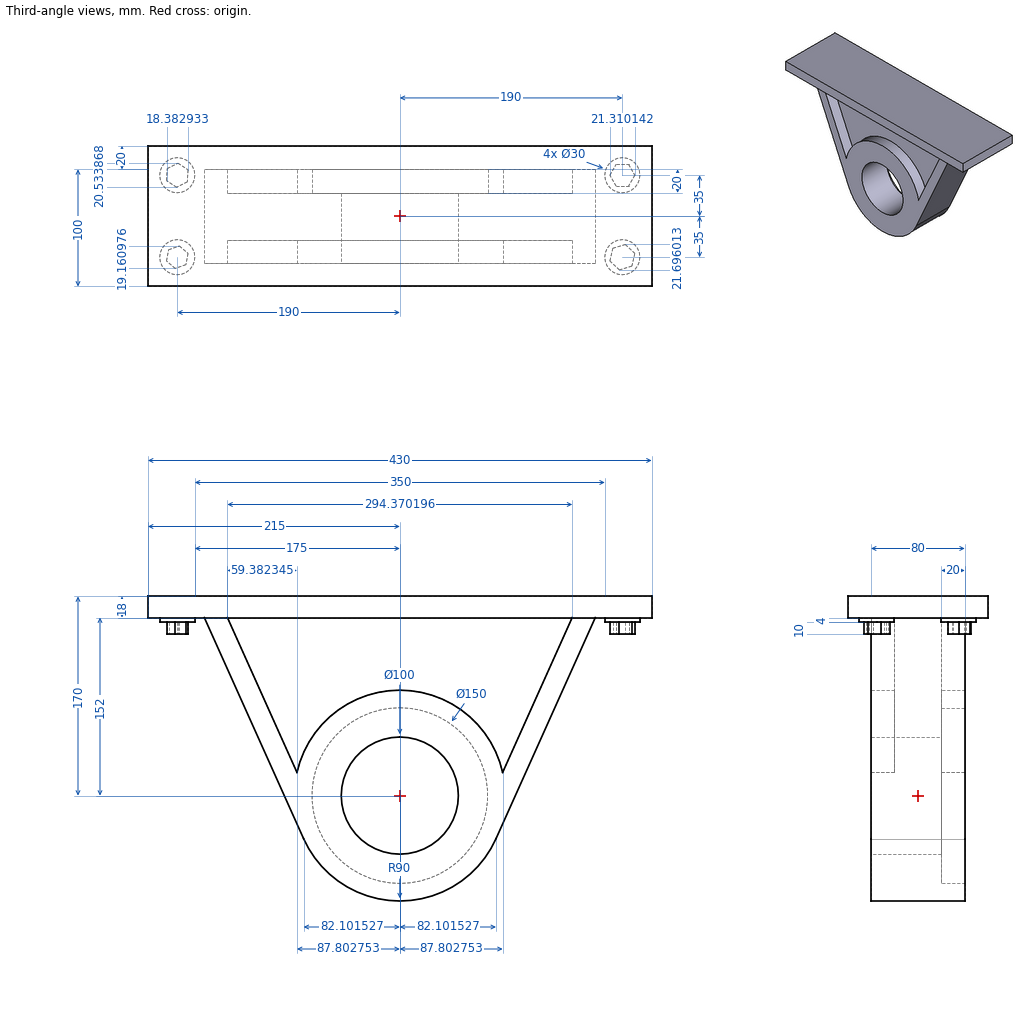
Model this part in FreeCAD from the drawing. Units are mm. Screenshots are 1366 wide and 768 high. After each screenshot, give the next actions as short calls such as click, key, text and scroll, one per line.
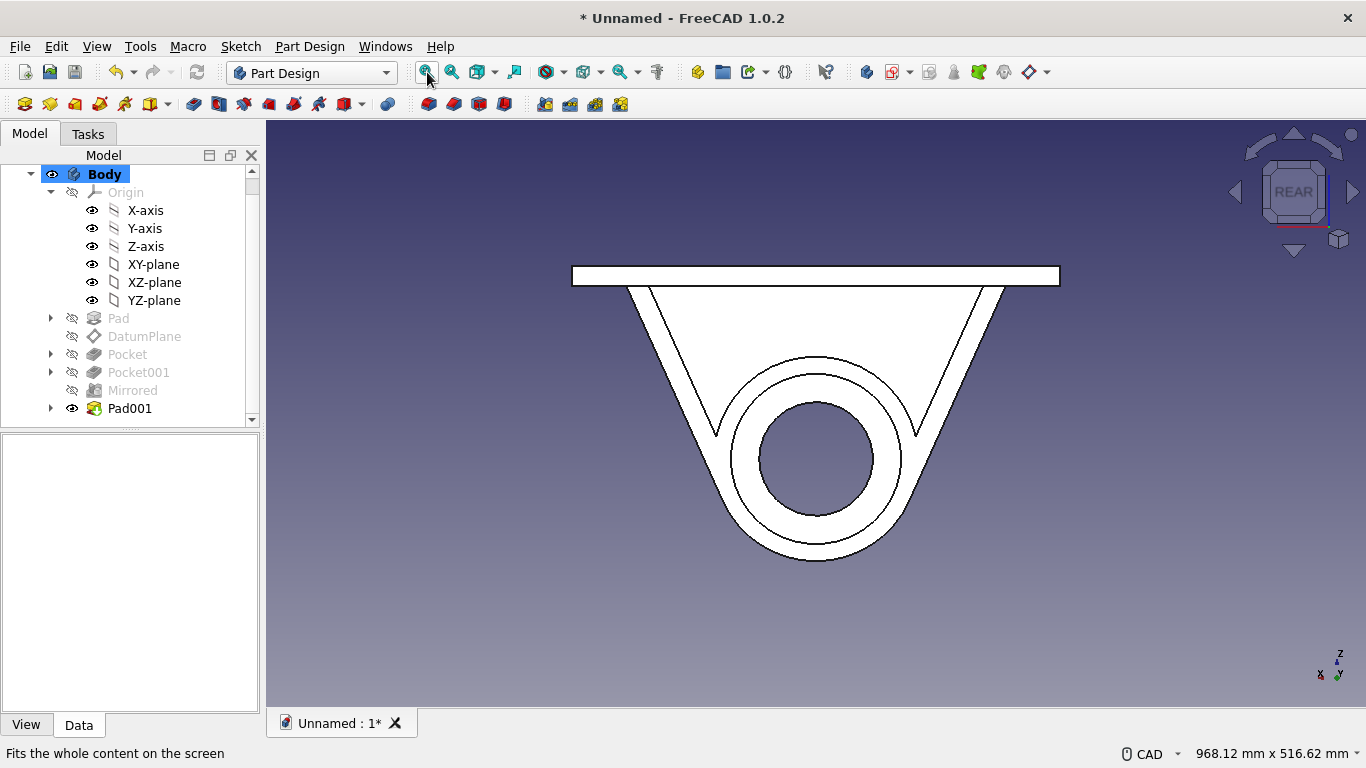
key(5)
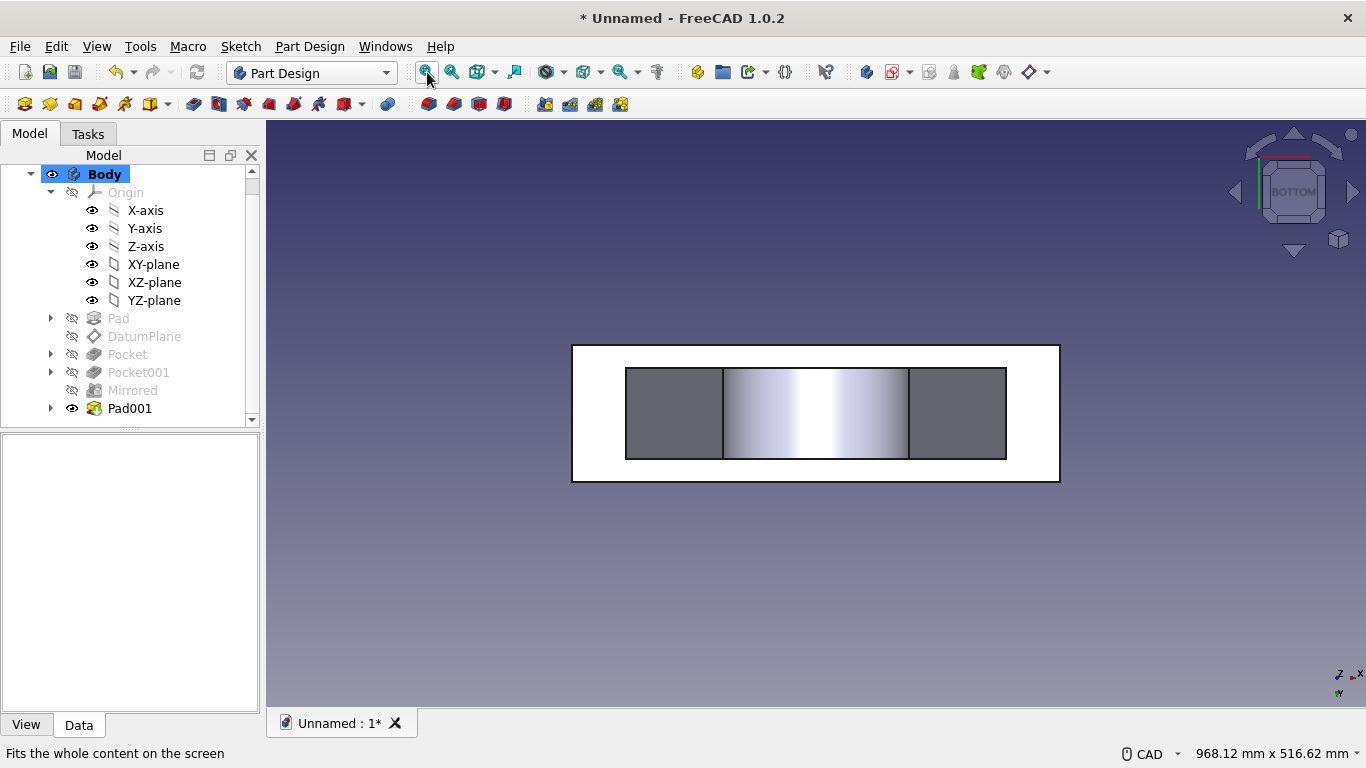
click(427, 72)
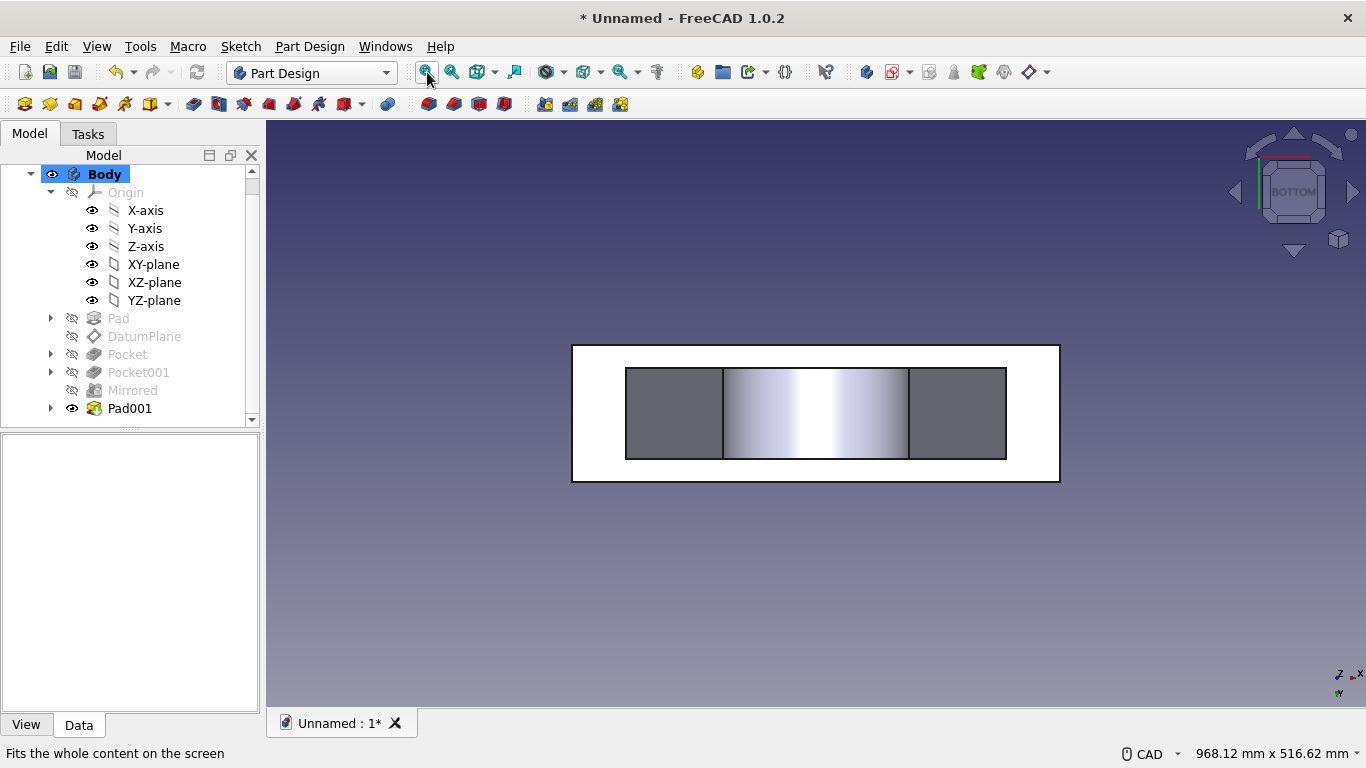
click(1025, 451)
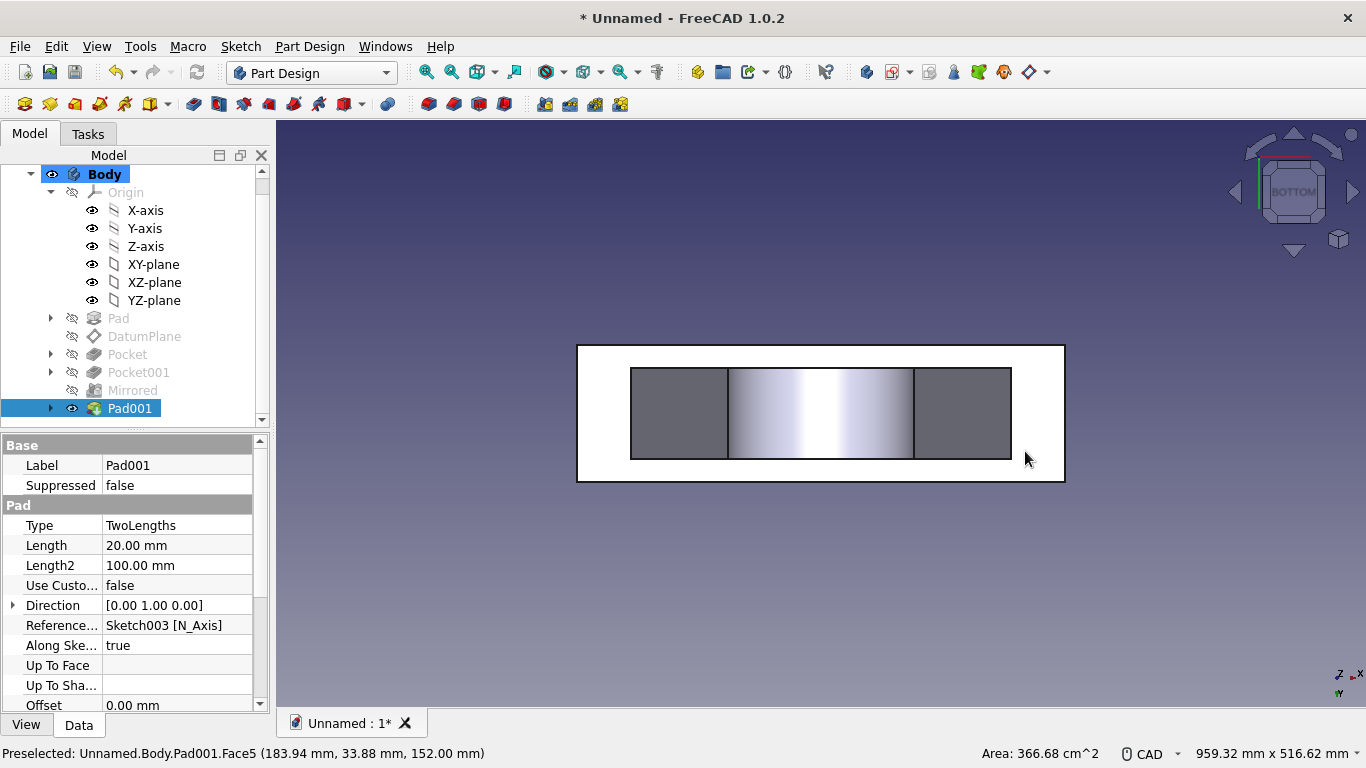
click(892, 72)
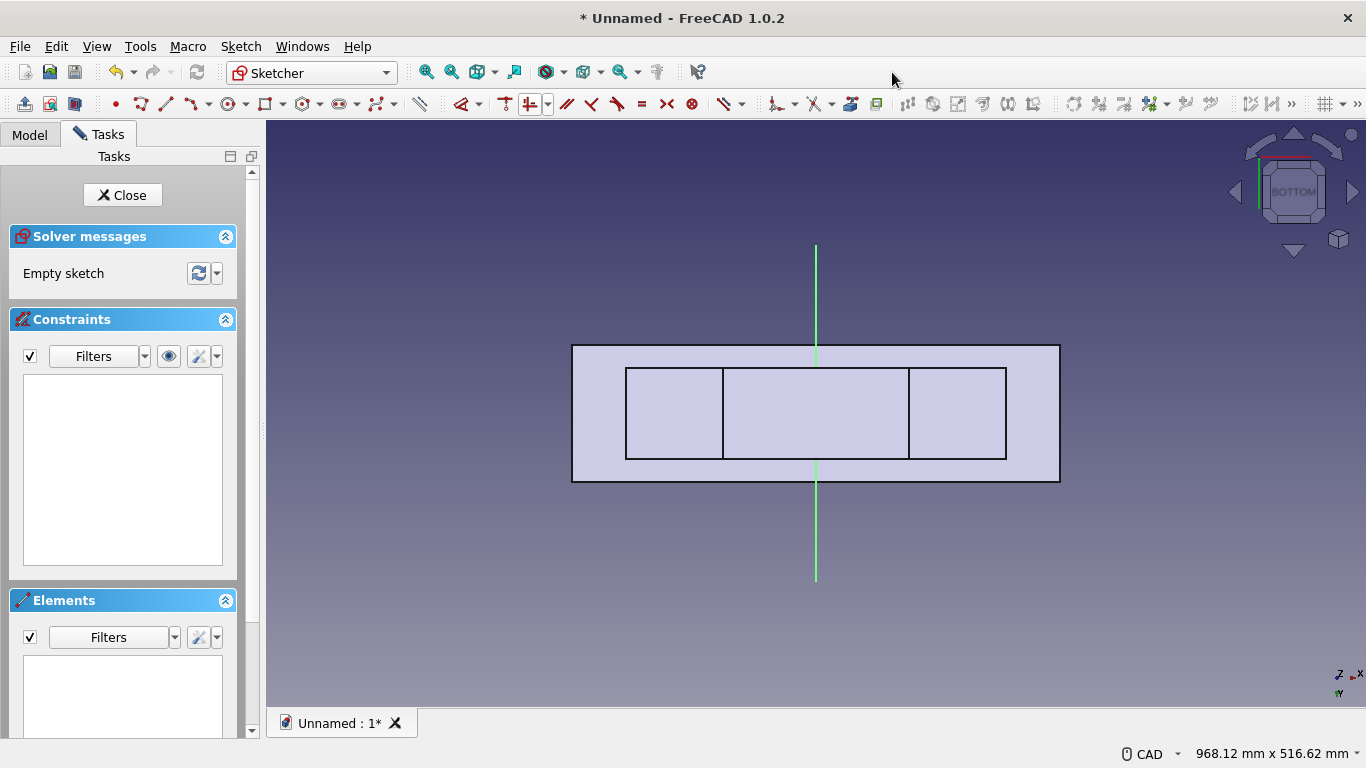
scroll(955, 414, up, 2)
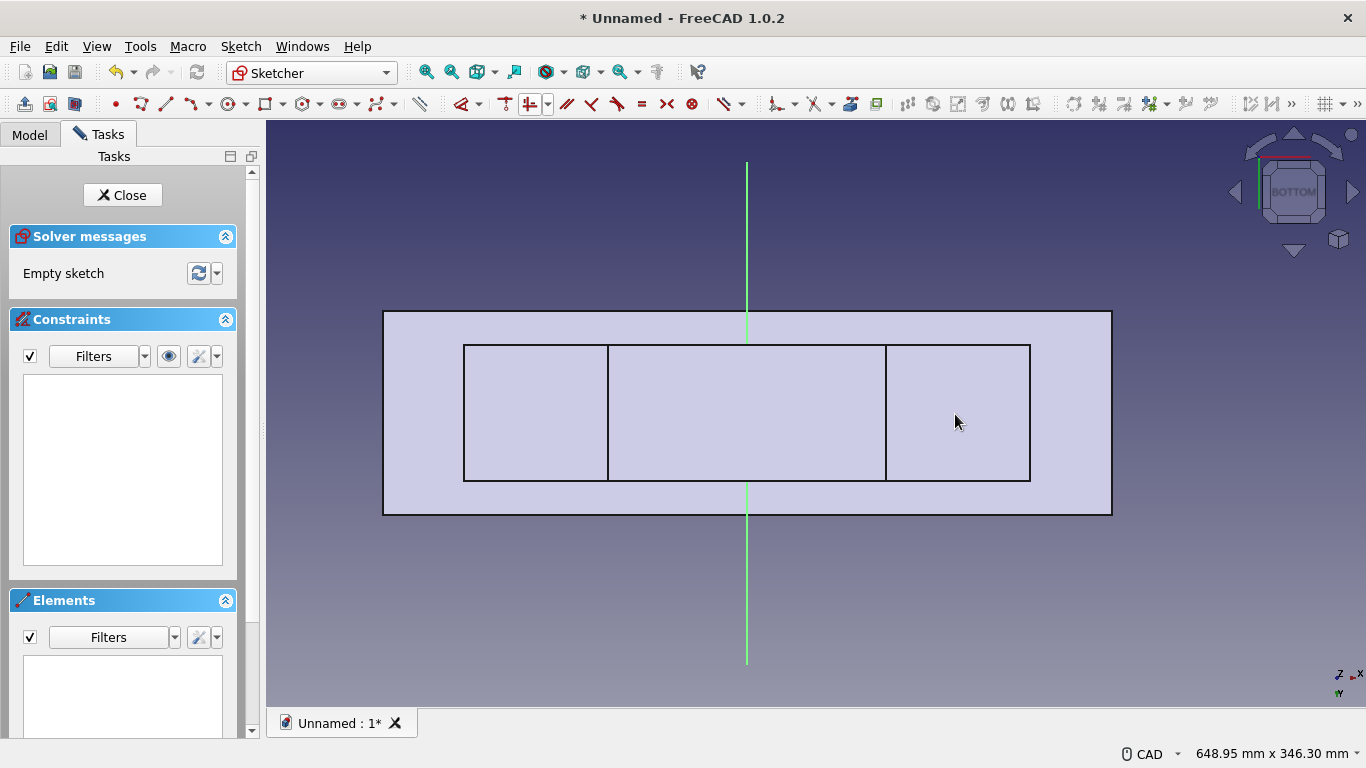
click(228, 104)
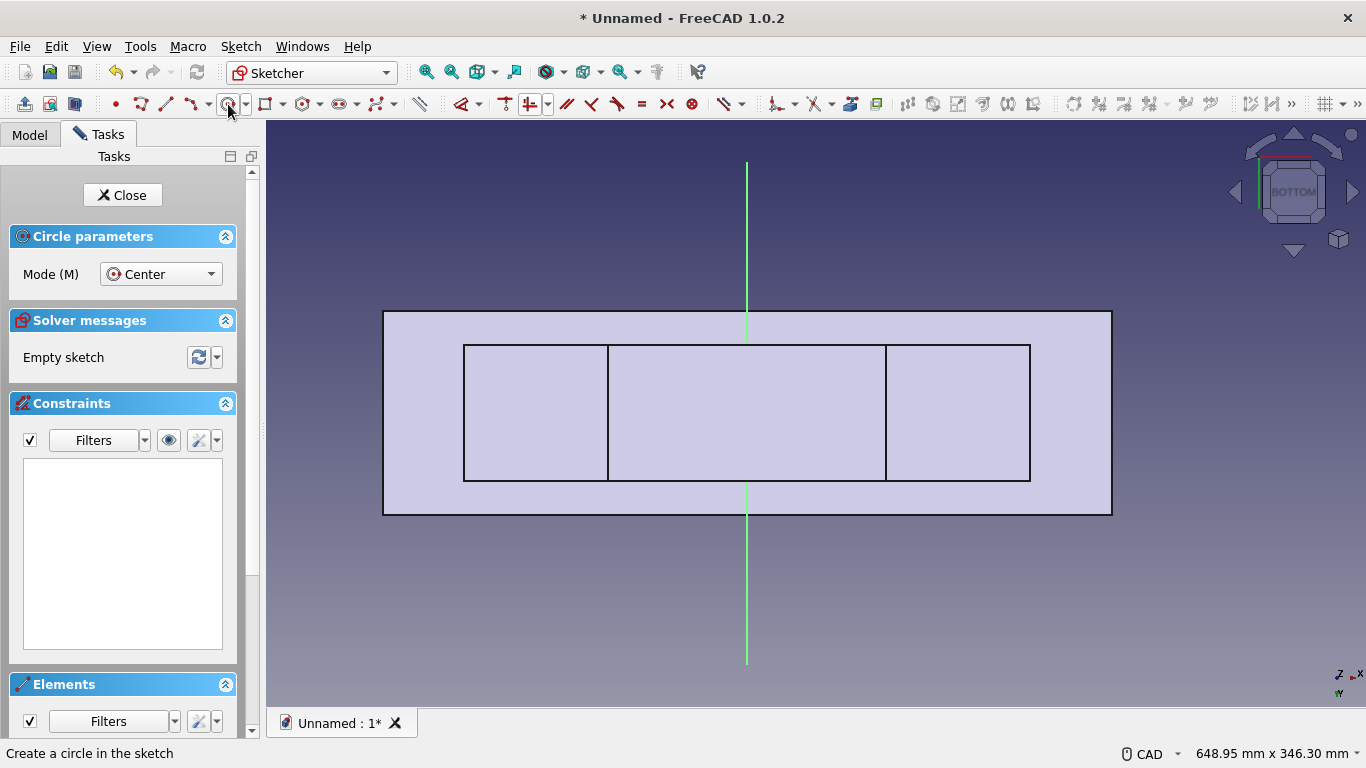
click(1069, 472)
click(1087, 454)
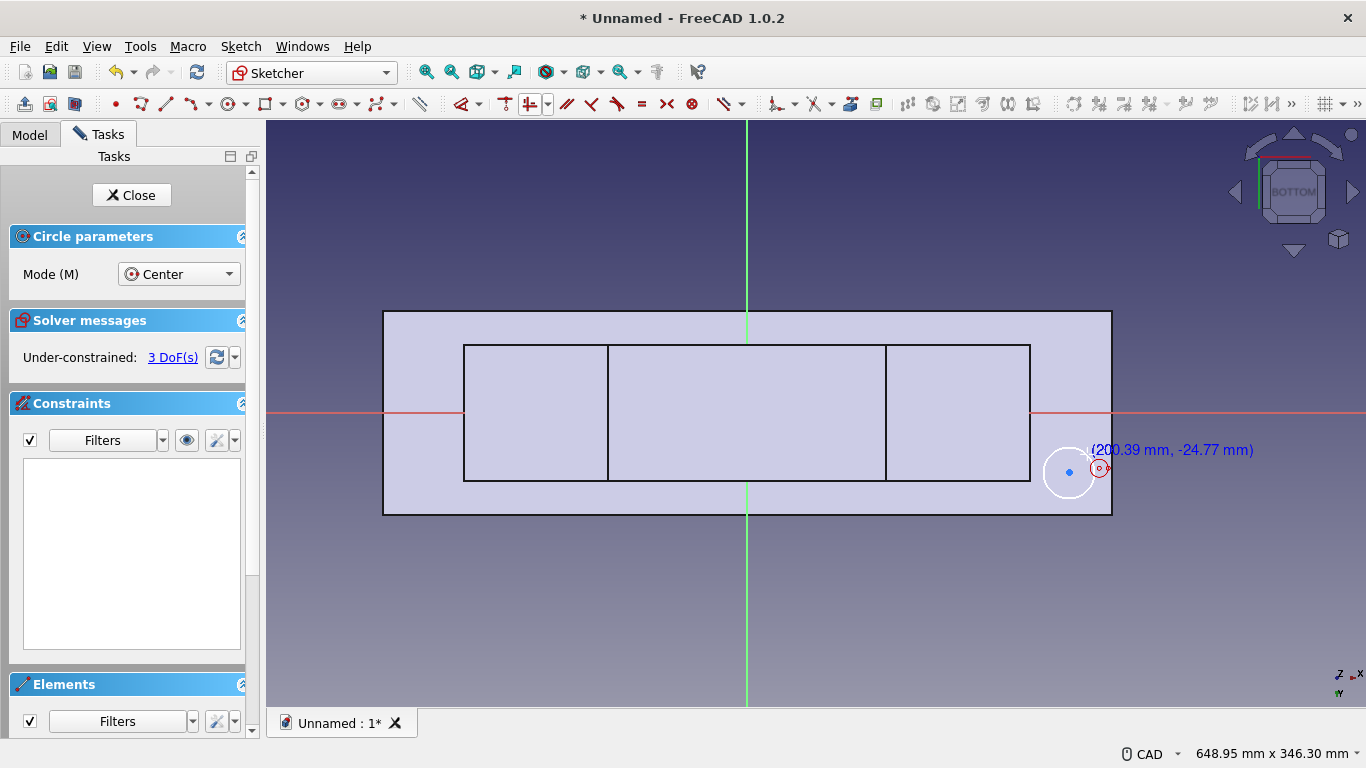
click(1069, 354)
click(1087, 336)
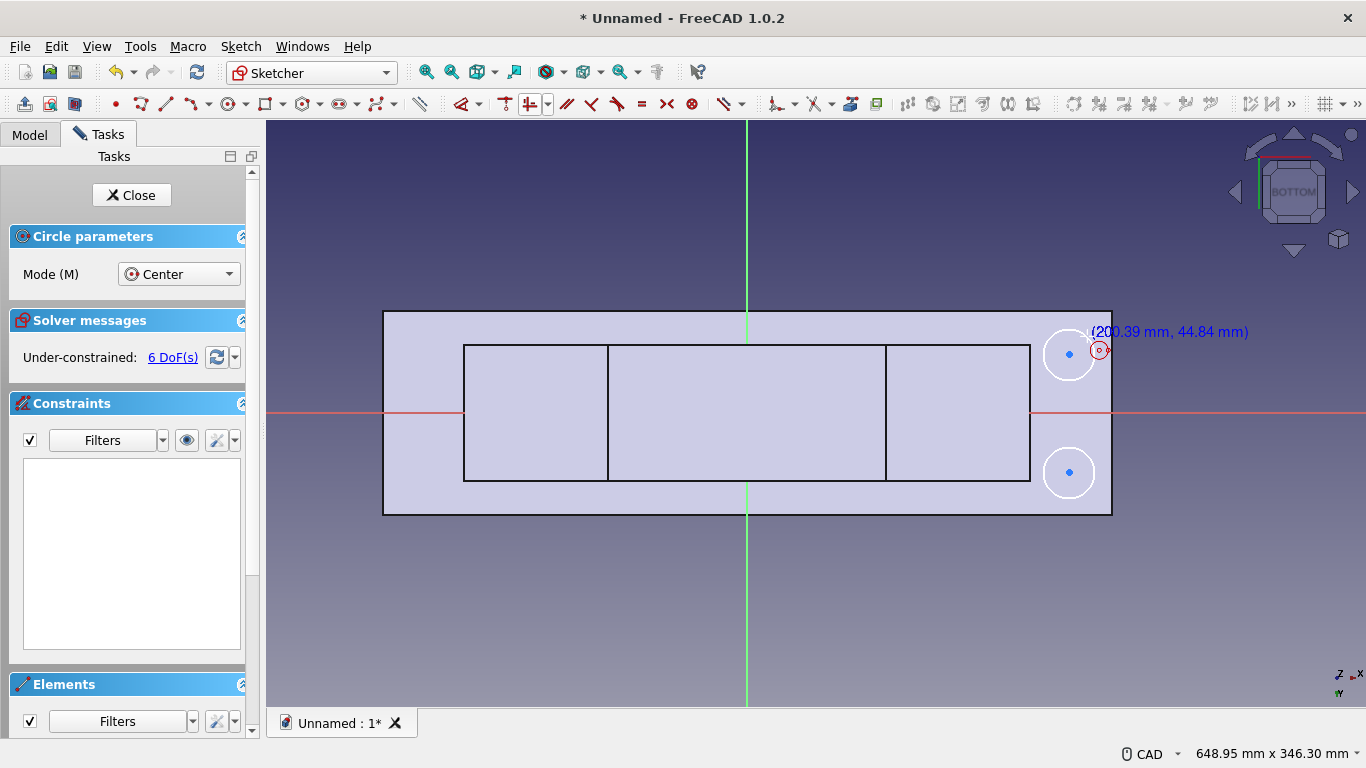
click(425, 354)
click(443, 336)